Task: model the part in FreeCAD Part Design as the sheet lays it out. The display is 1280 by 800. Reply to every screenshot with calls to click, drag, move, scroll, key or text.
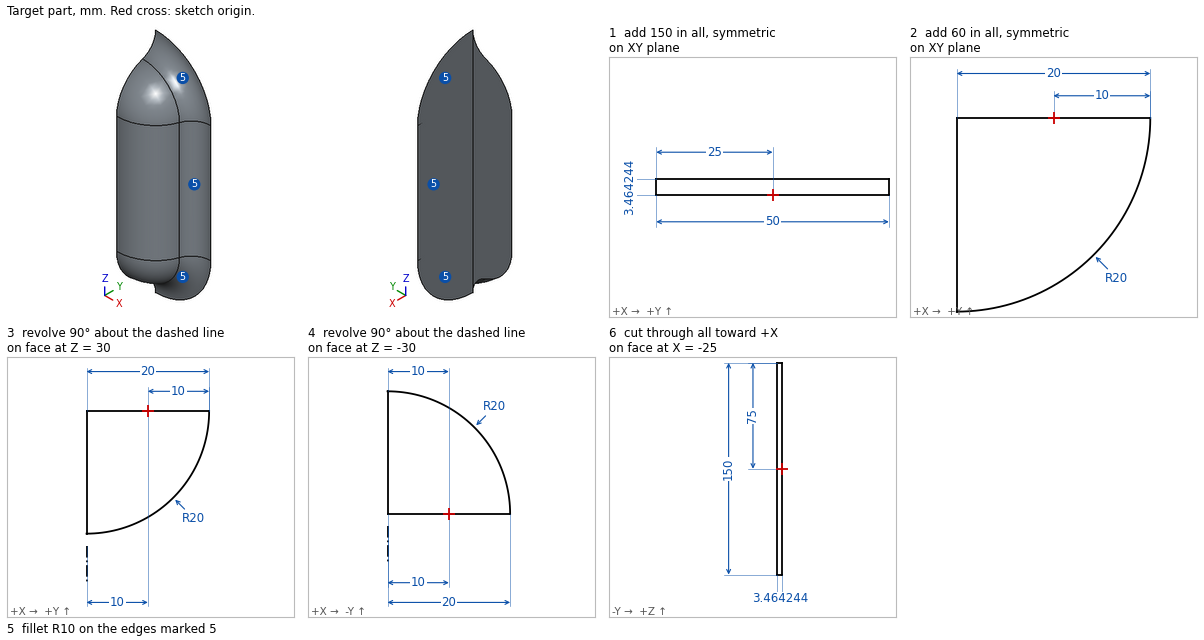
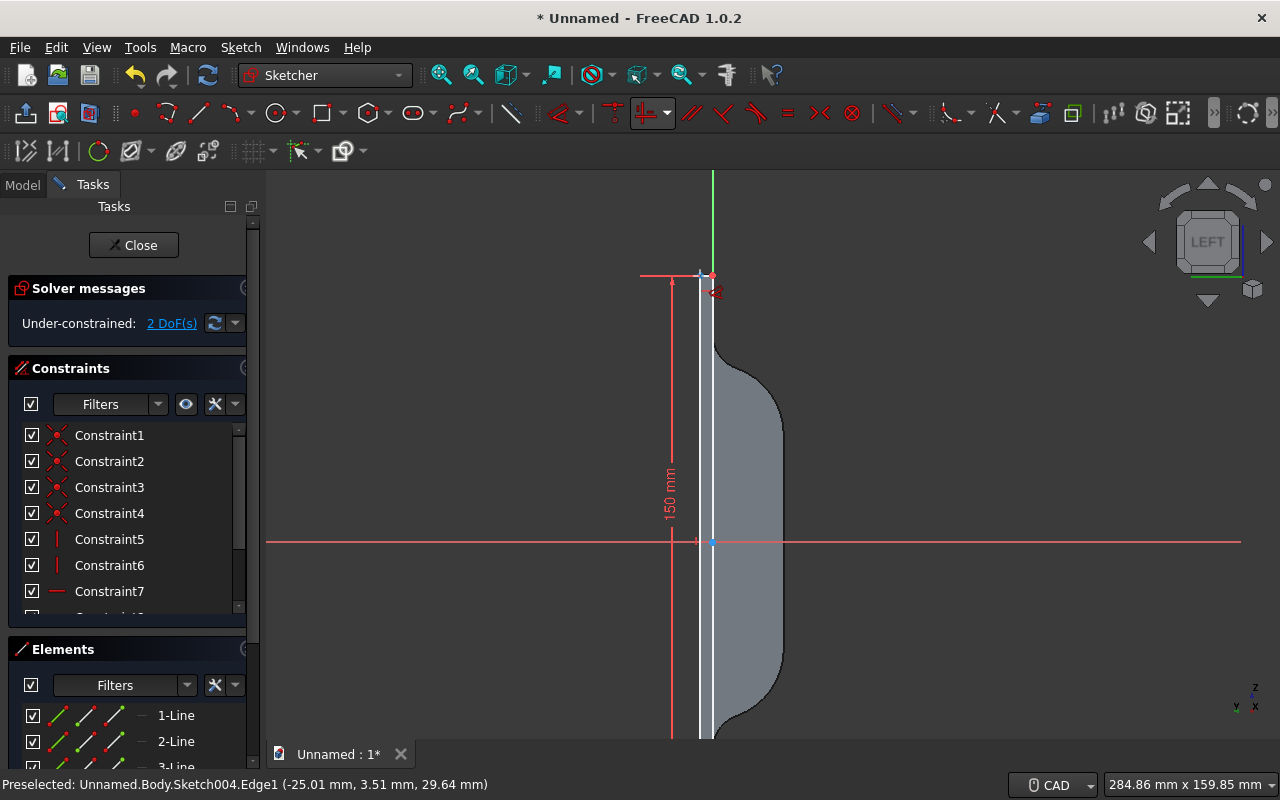
click(700, 276)
click(666, 409)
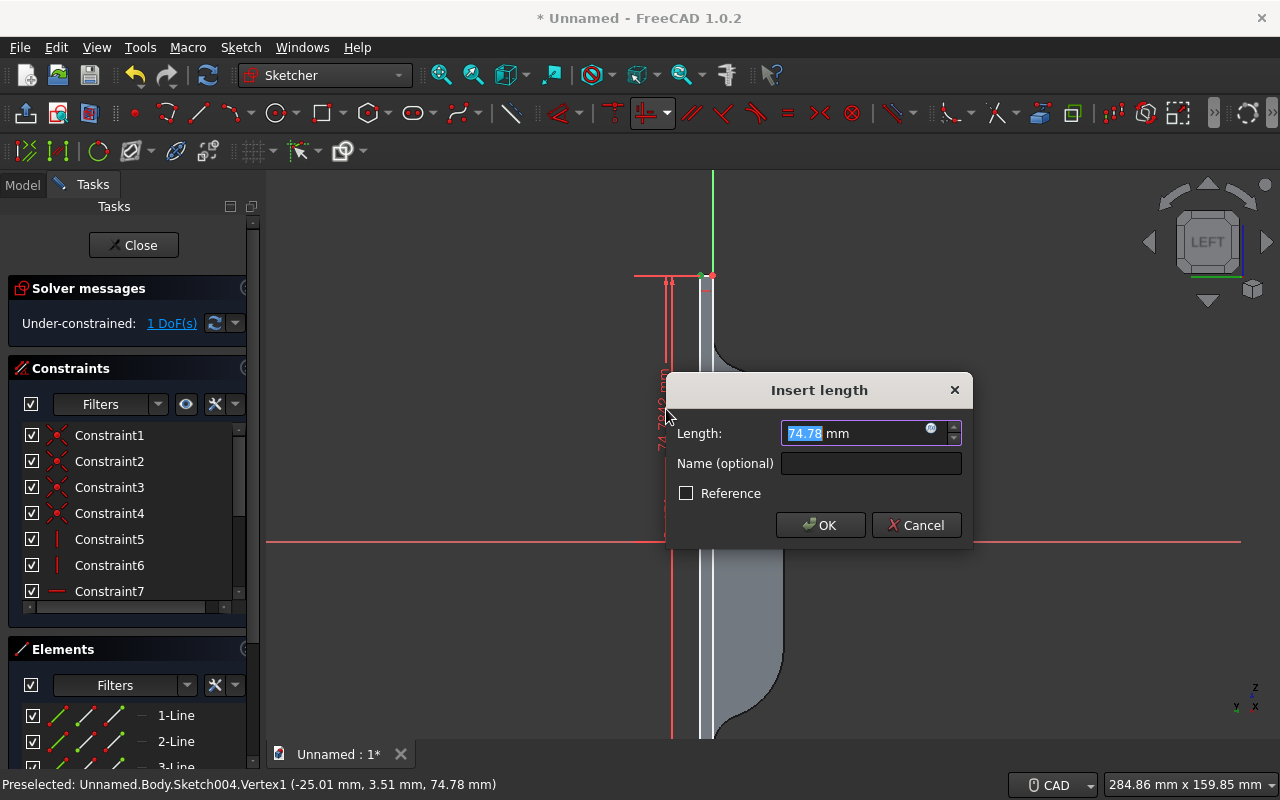
text(75)
key(Return)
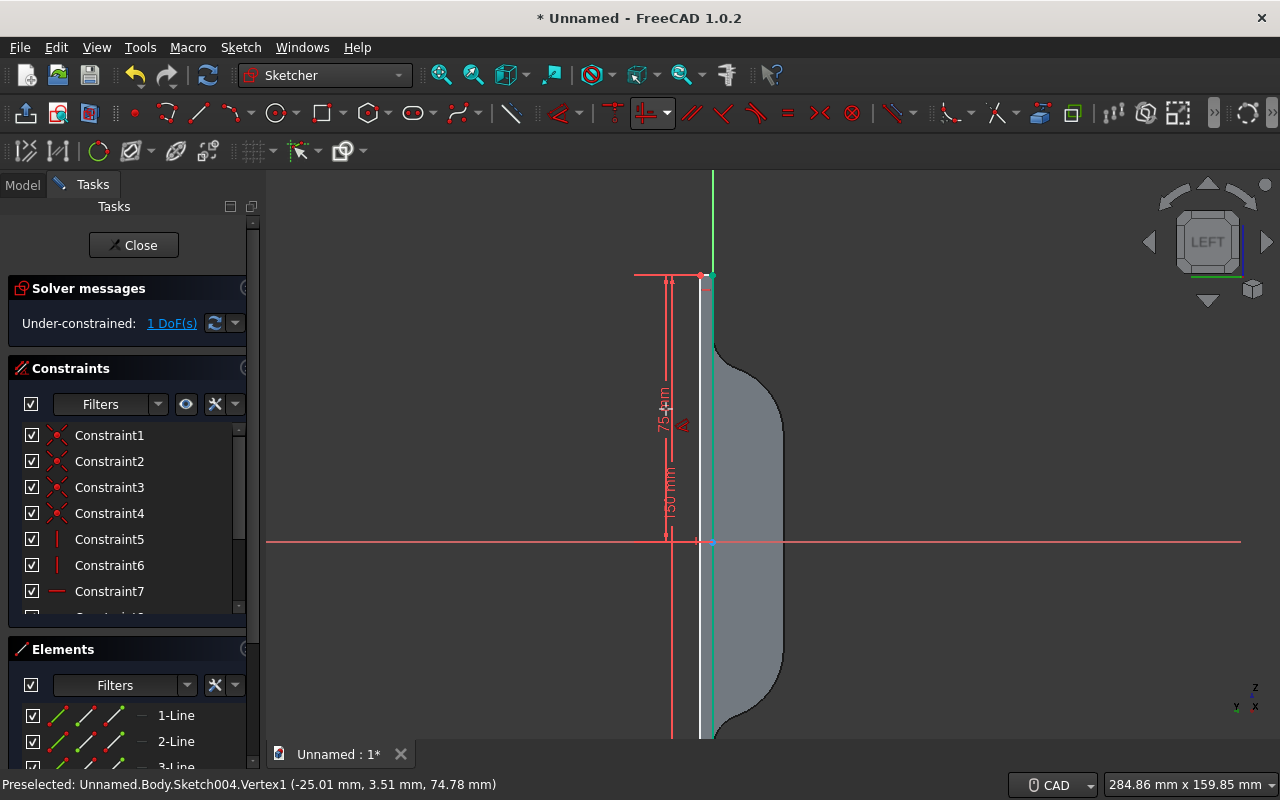
scroll(700, 276, down, 2)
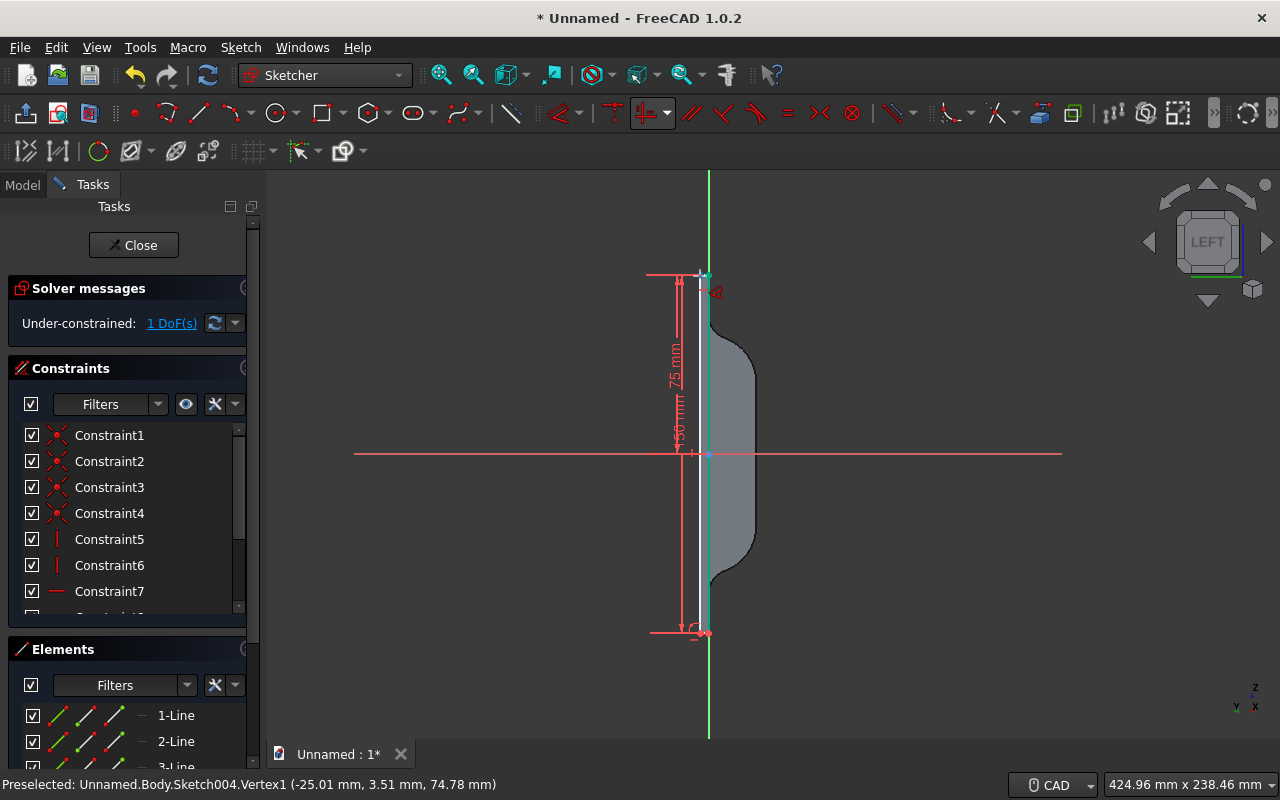
scroll(704, 633, up, 8)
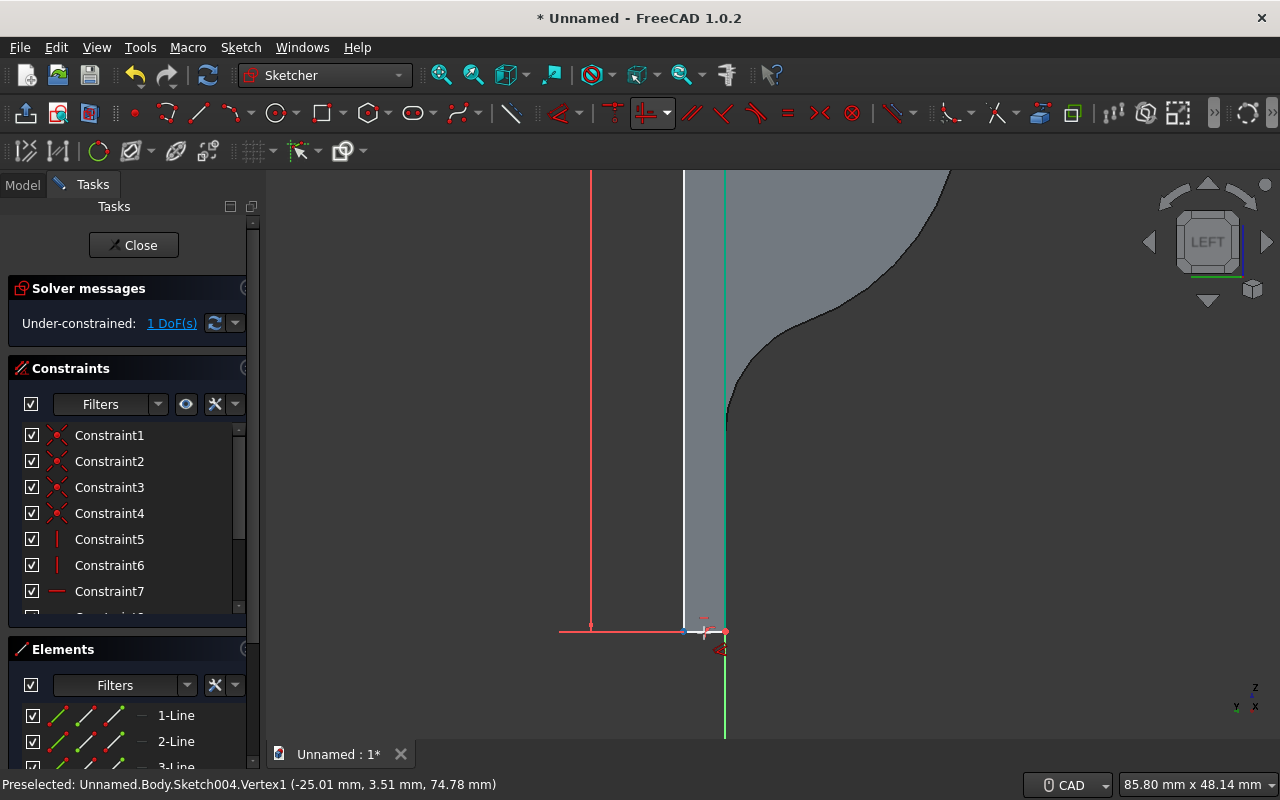
click(704, 632)
click(704, 666)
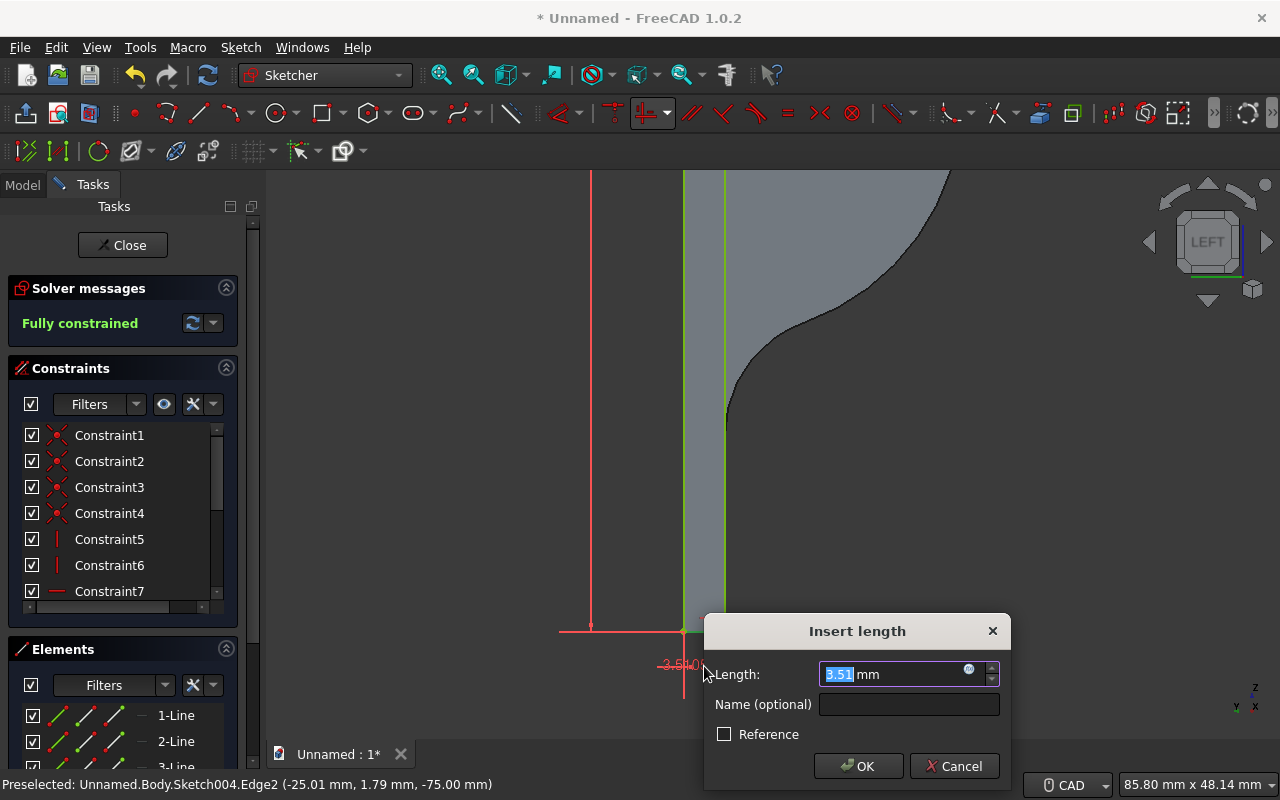
text(3.464244)
key(Return)
key(Escape)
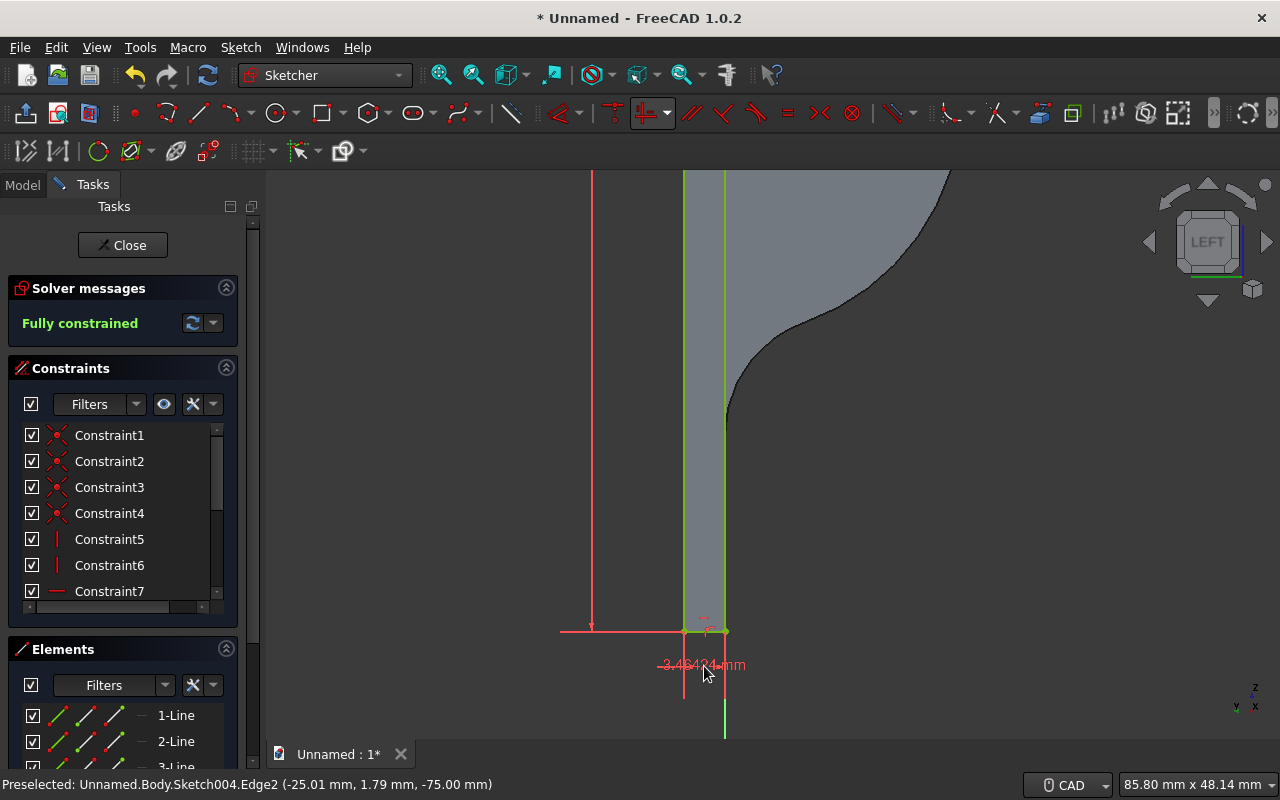
click(123, 245)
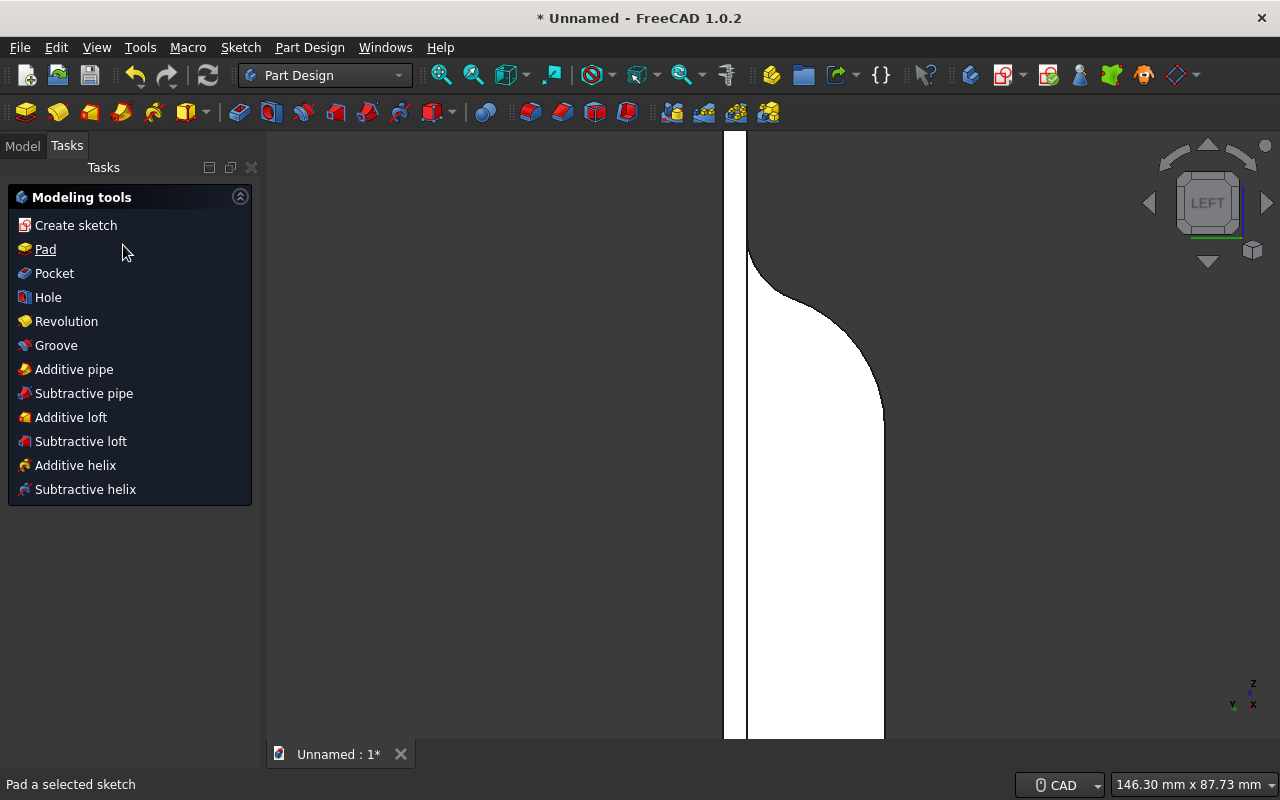
click(240, 112)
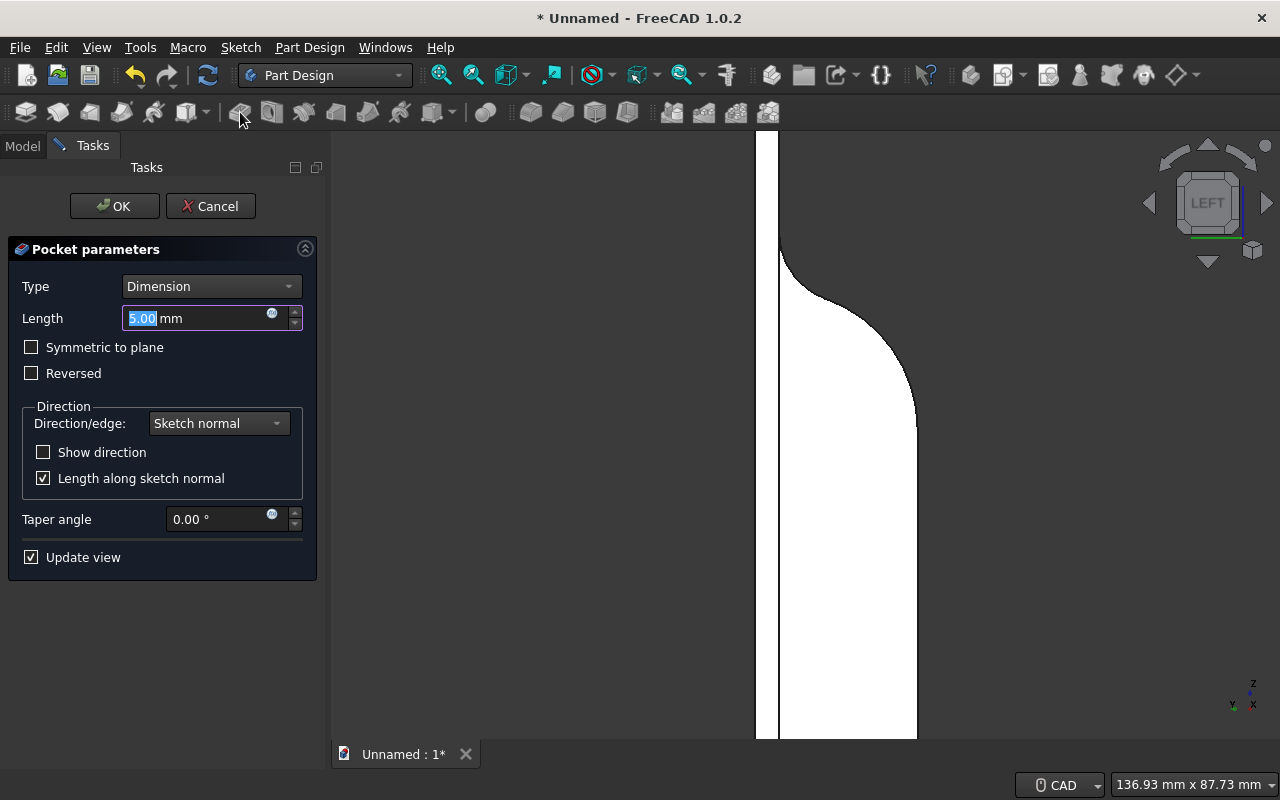
click(212, 286)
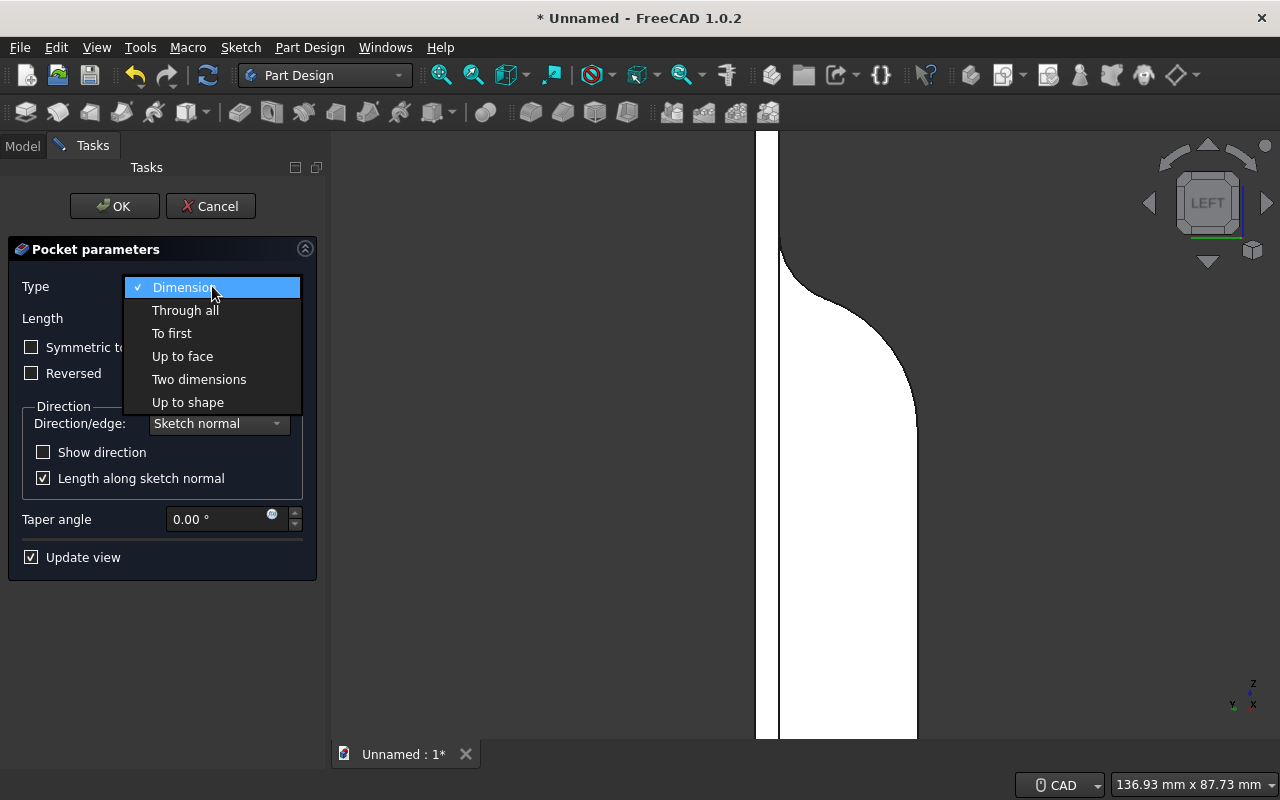
click(212, 310)